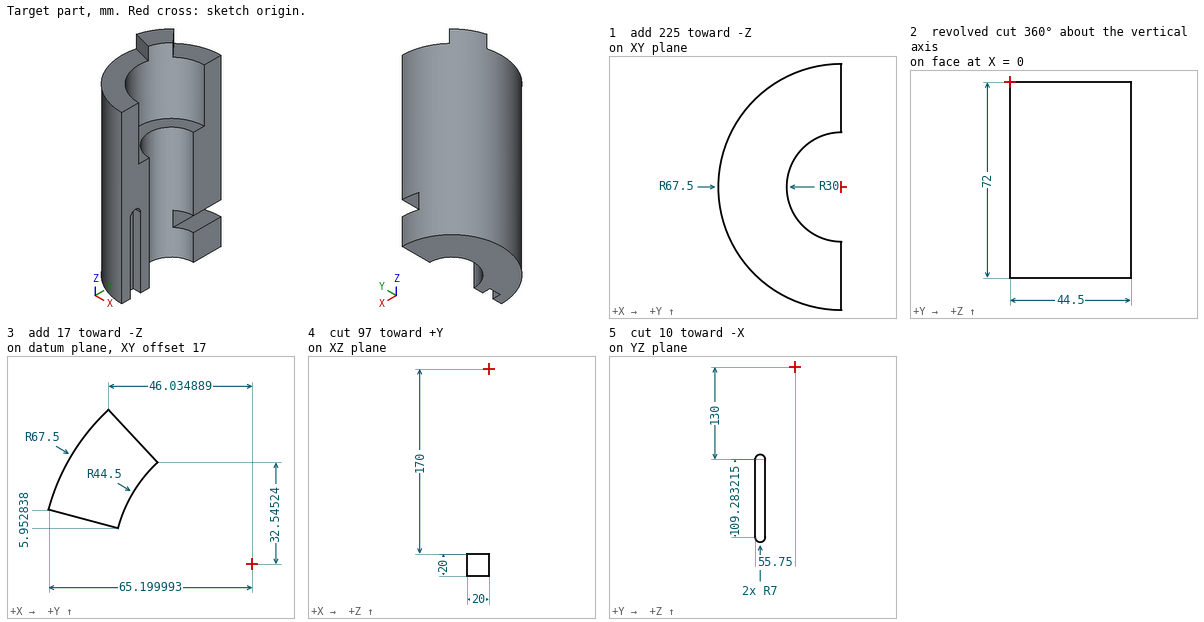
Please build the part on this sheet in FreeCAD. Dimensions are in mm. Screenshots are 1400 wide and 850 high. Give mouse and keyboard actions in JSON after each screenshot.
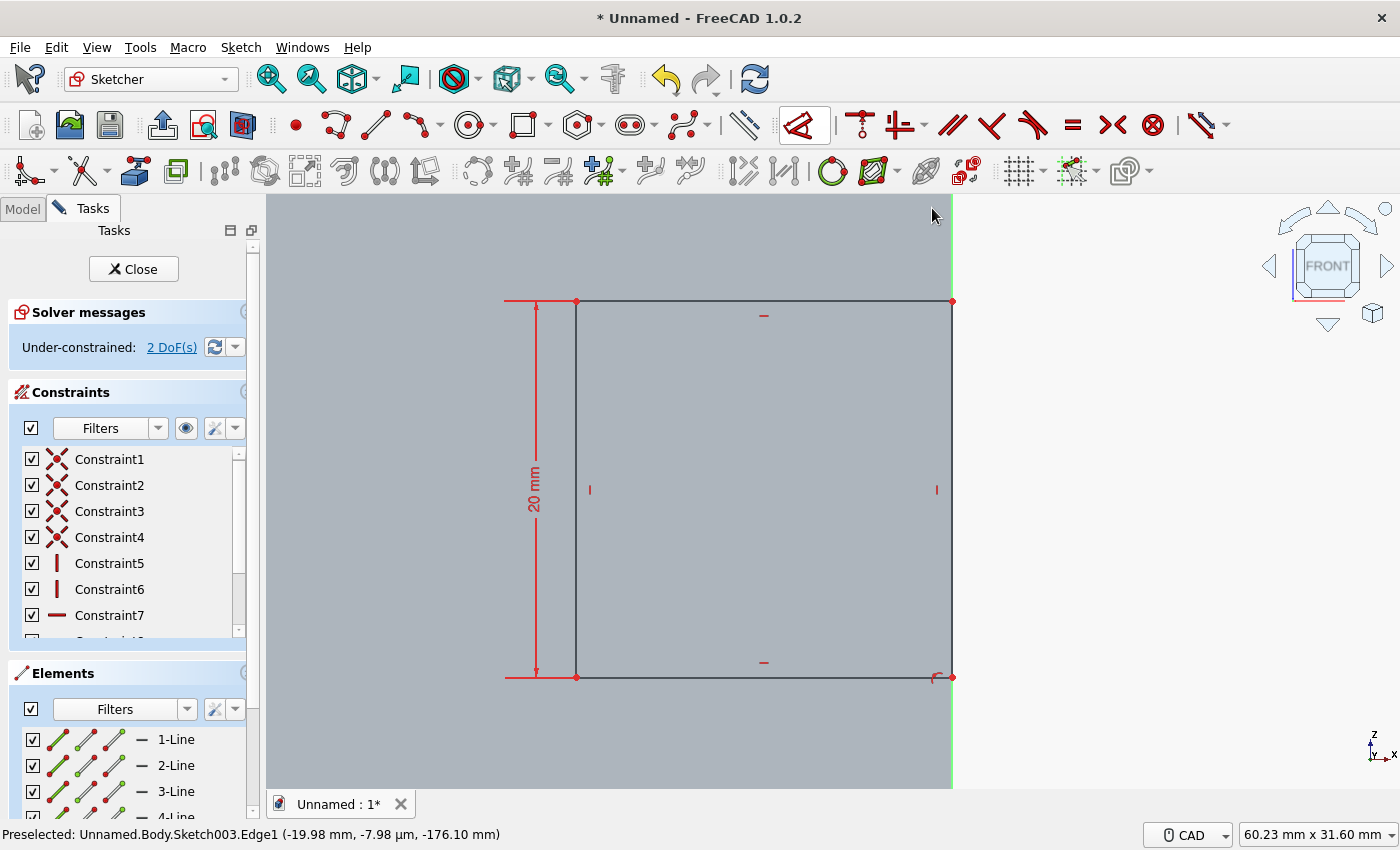
{"action": "left_click", "coordinate": [689, 678]}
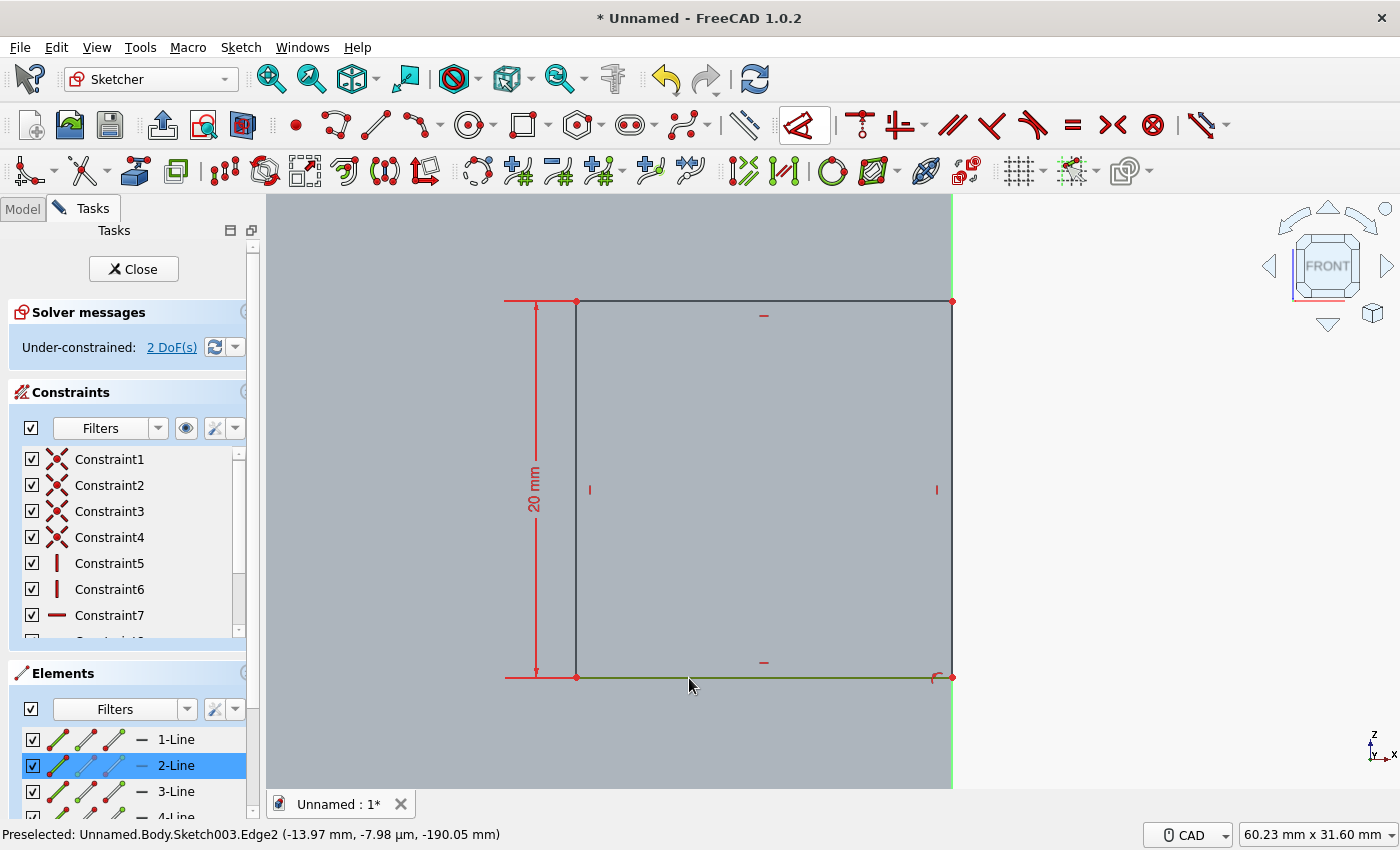
{"action": "key", "text": "l"}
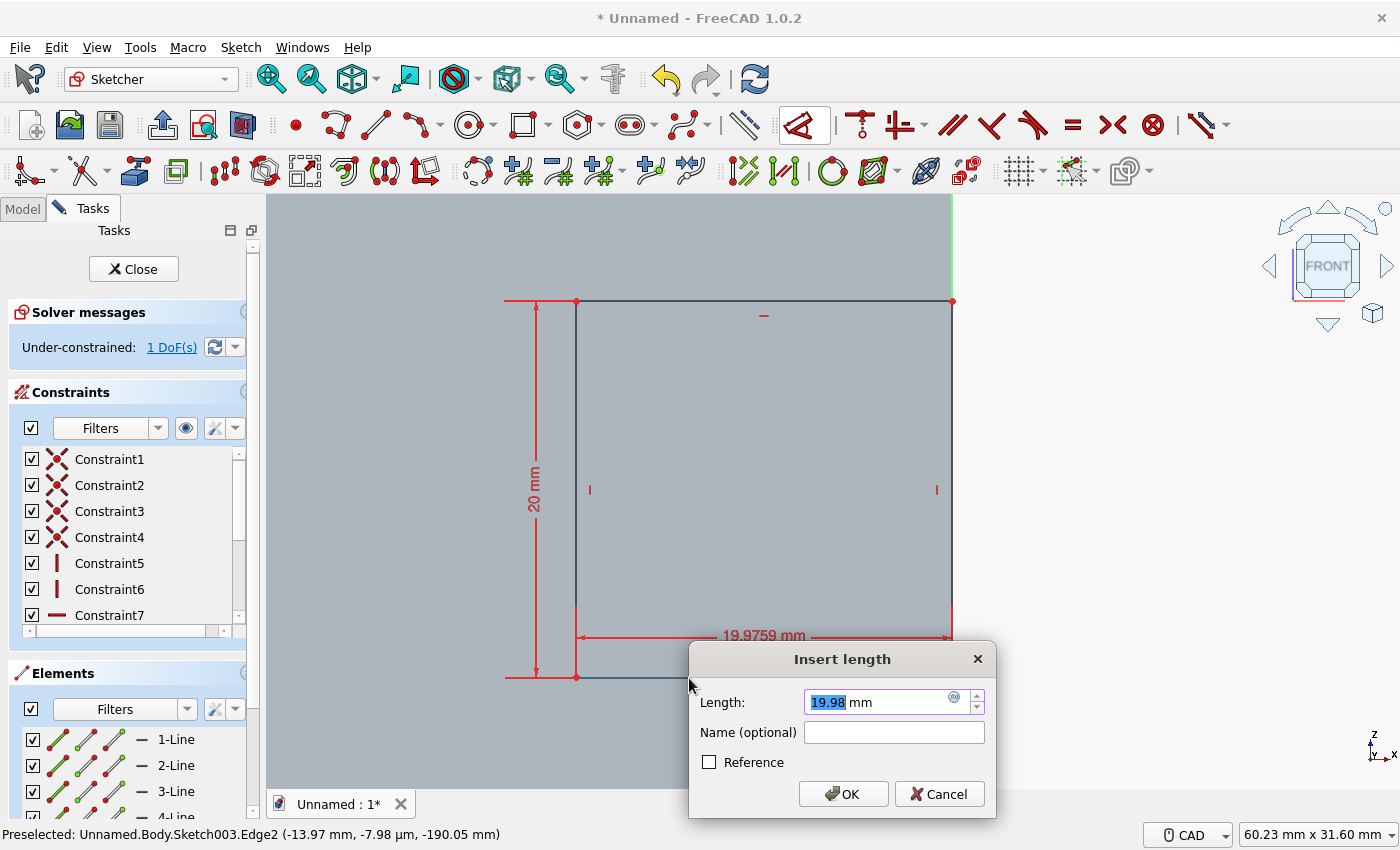
{"action": "type", "text": "20"}
{"action": "key", "text": "Return"}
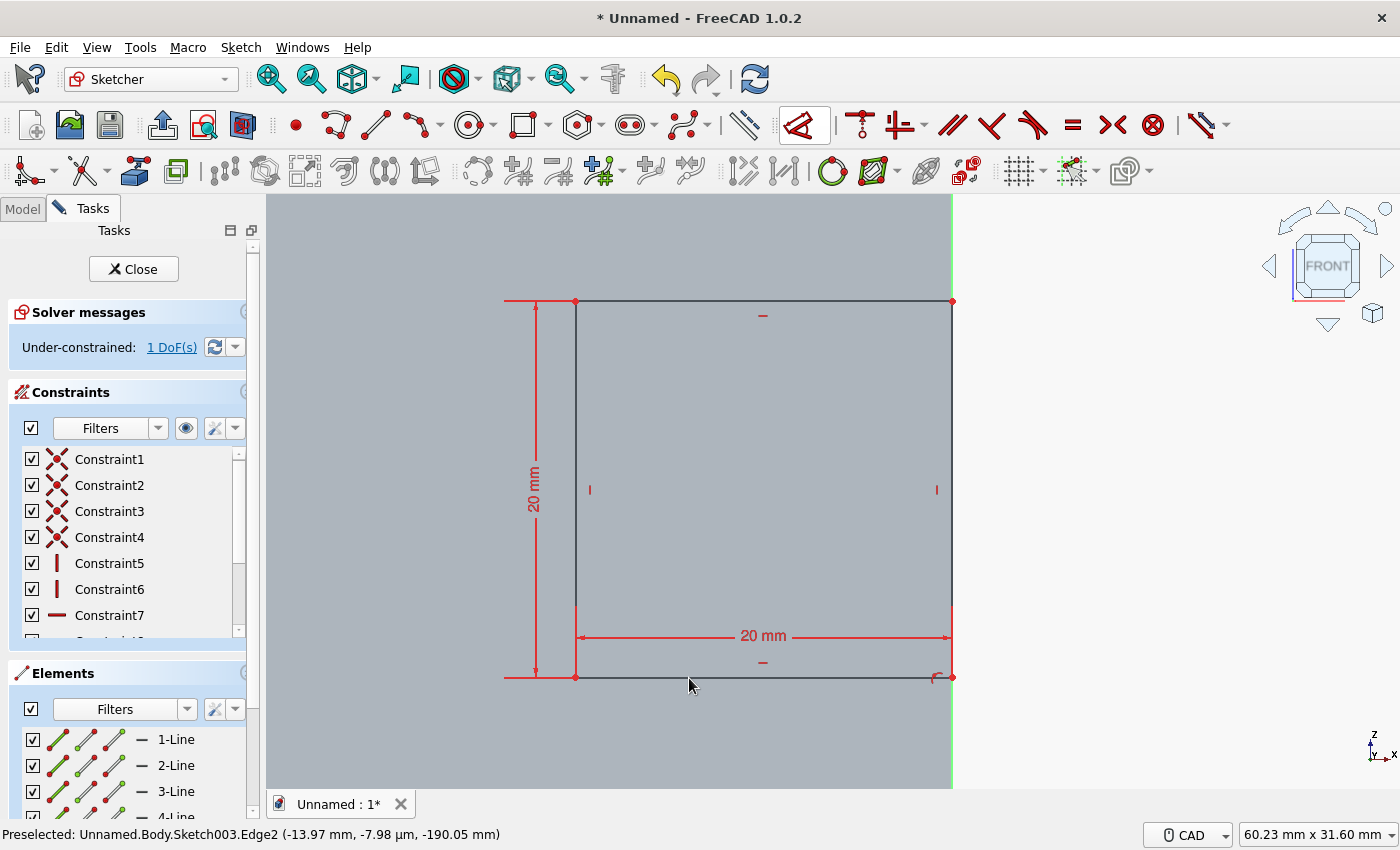
{"action": "left_click", "coordinate": [576, 301]}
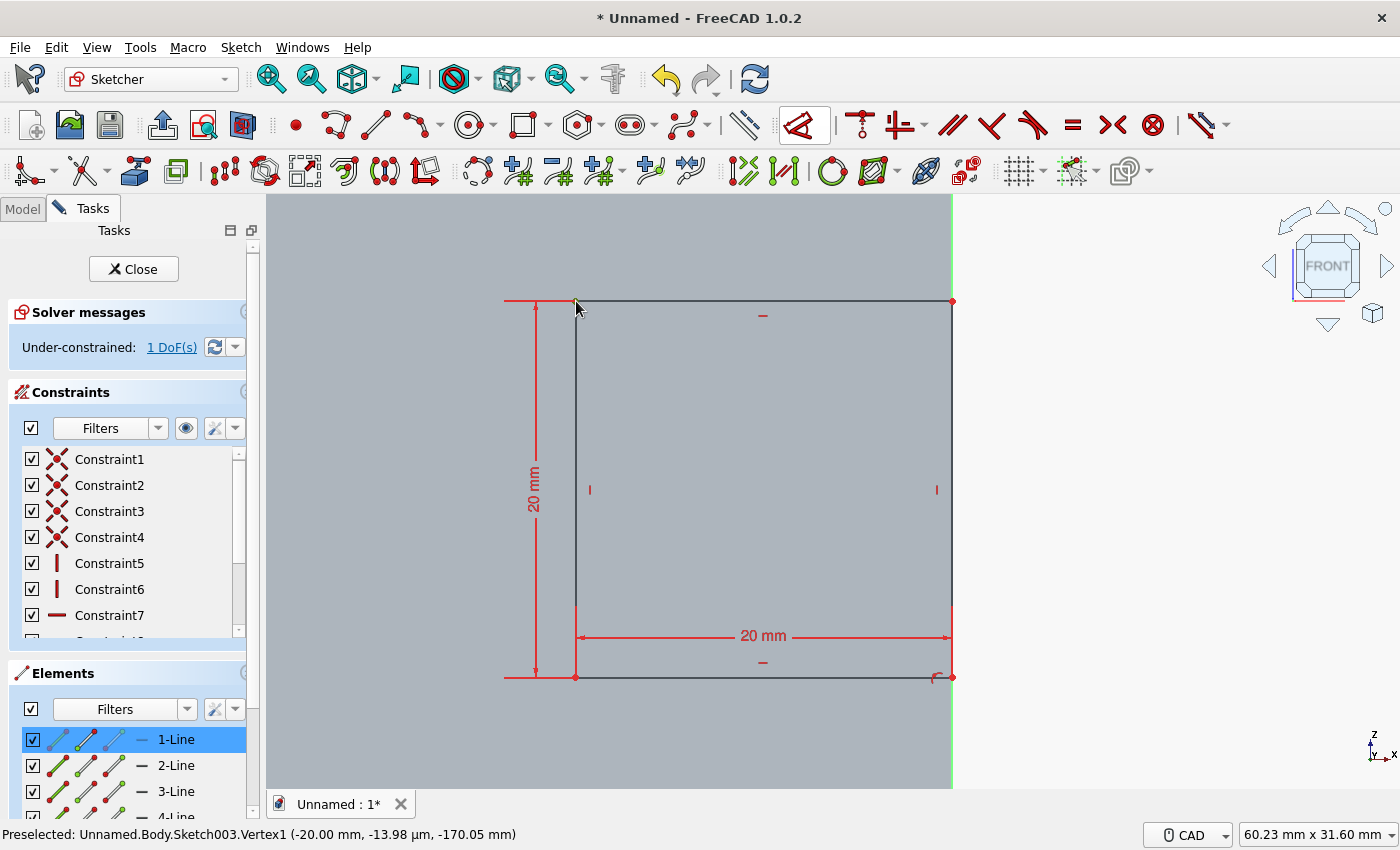
{"action": "key", "text": "i"}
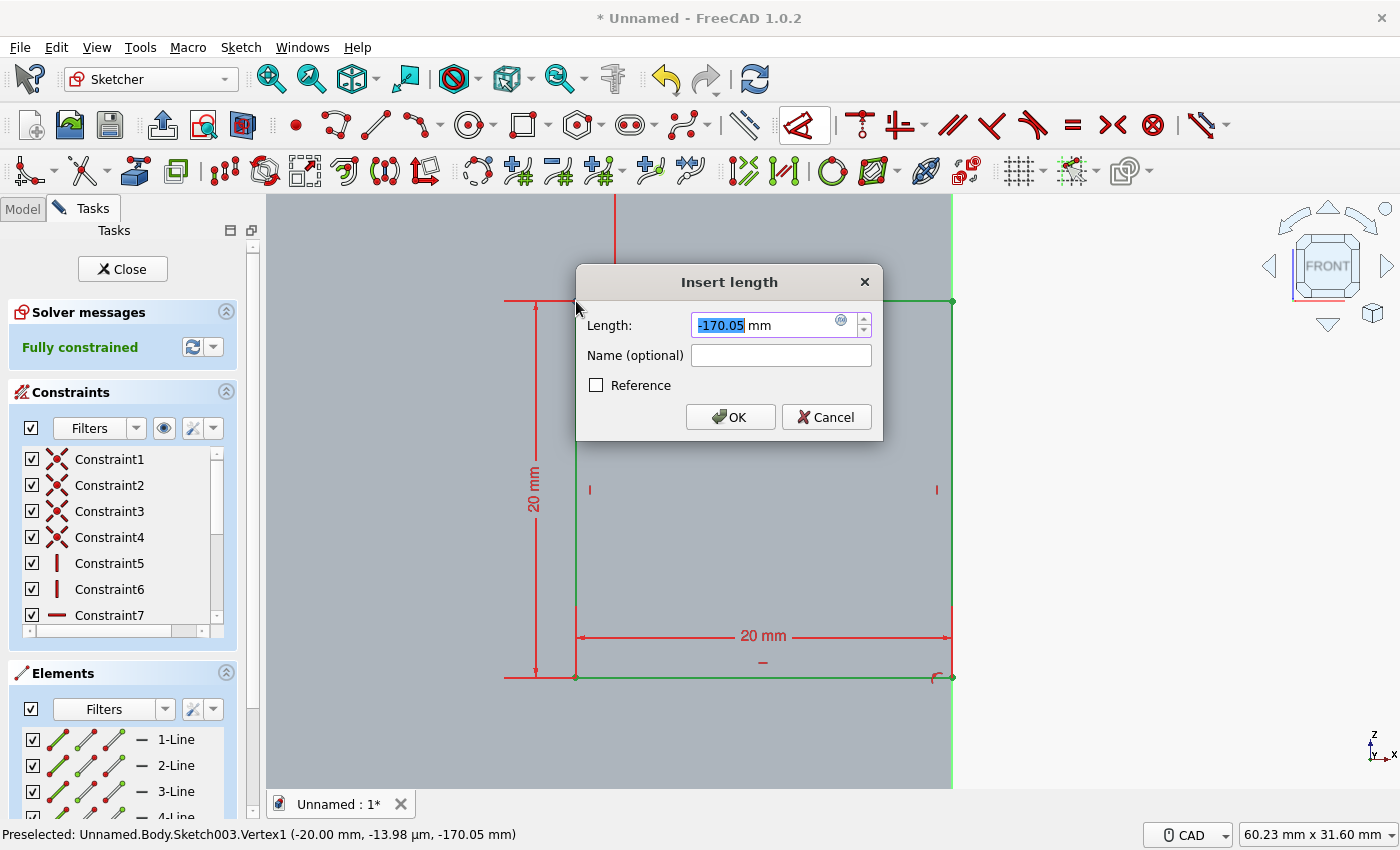
{"action": "type", "text": "-170"}
{"action": "key", "text": "Return"}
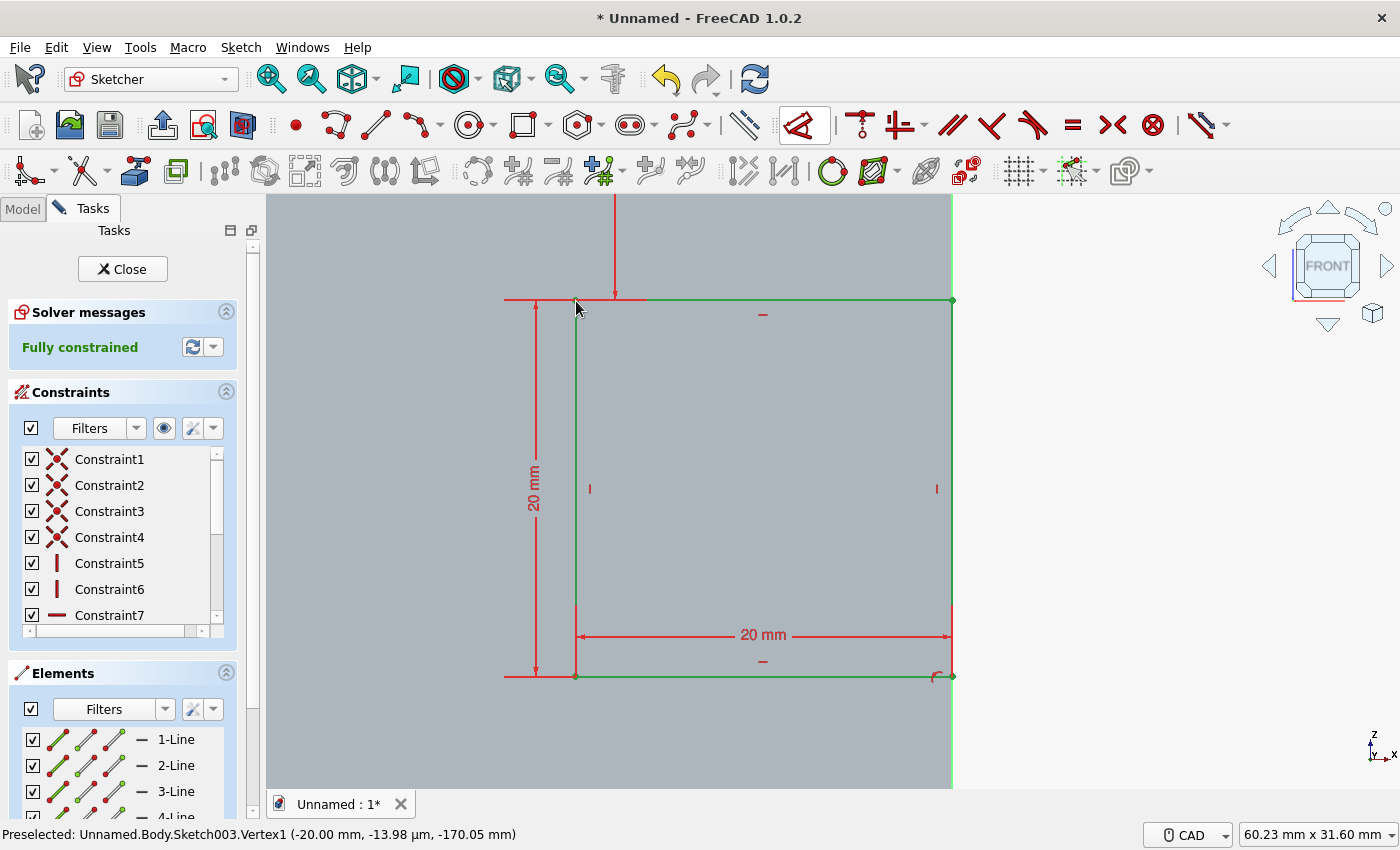
{"action": "left_click", "coordinate": [123, 269]}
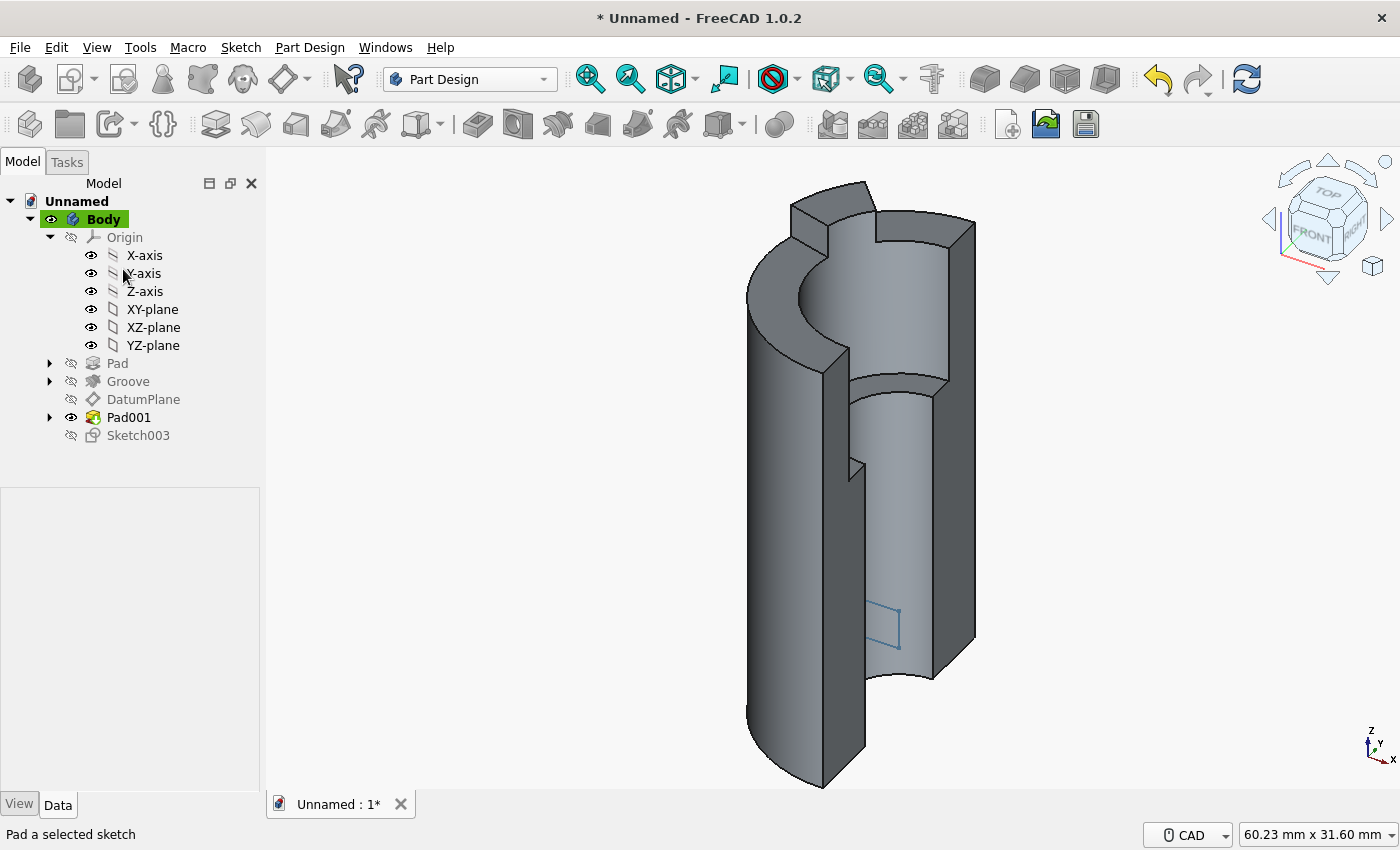
{"action": "left_click", "coordinate": [478, 124]}